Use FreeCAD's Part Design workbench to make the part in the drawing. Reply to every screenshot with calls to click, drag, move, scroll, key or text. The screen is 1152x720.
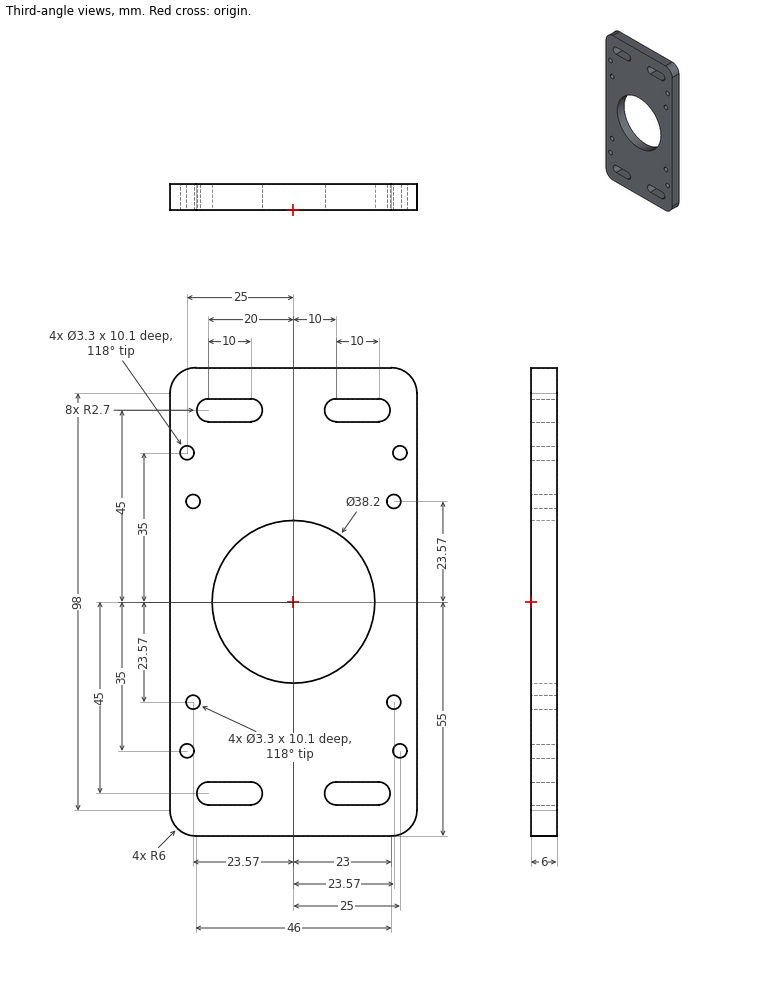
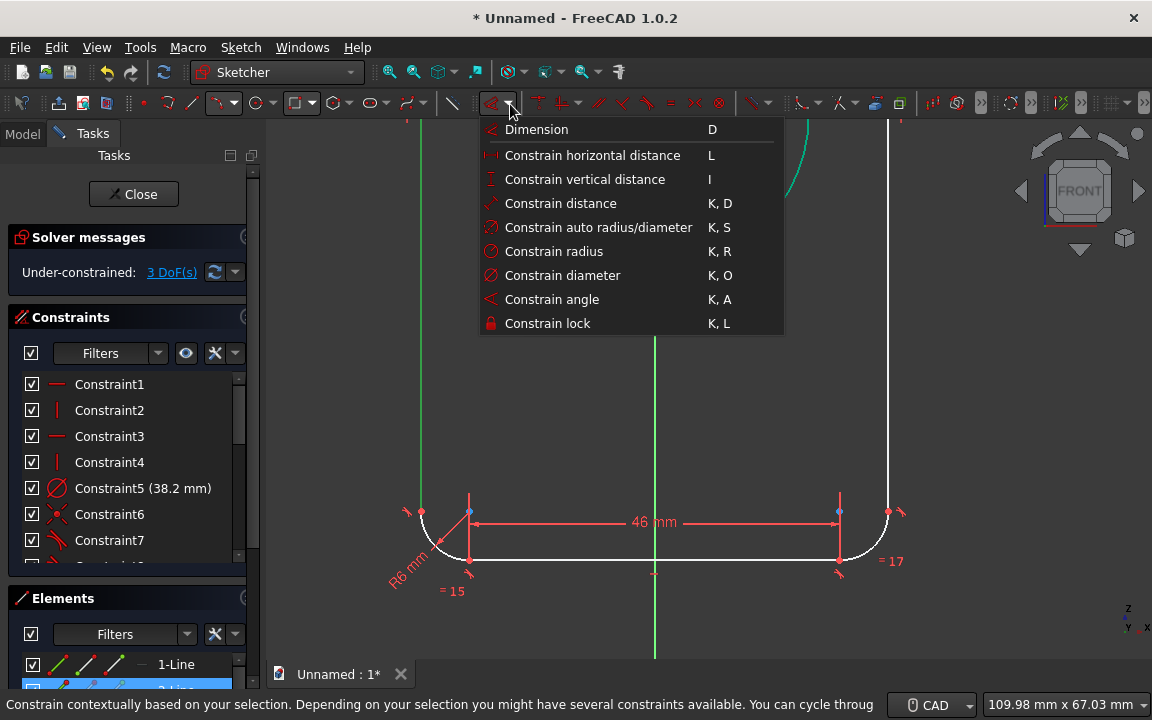
click(632, 179)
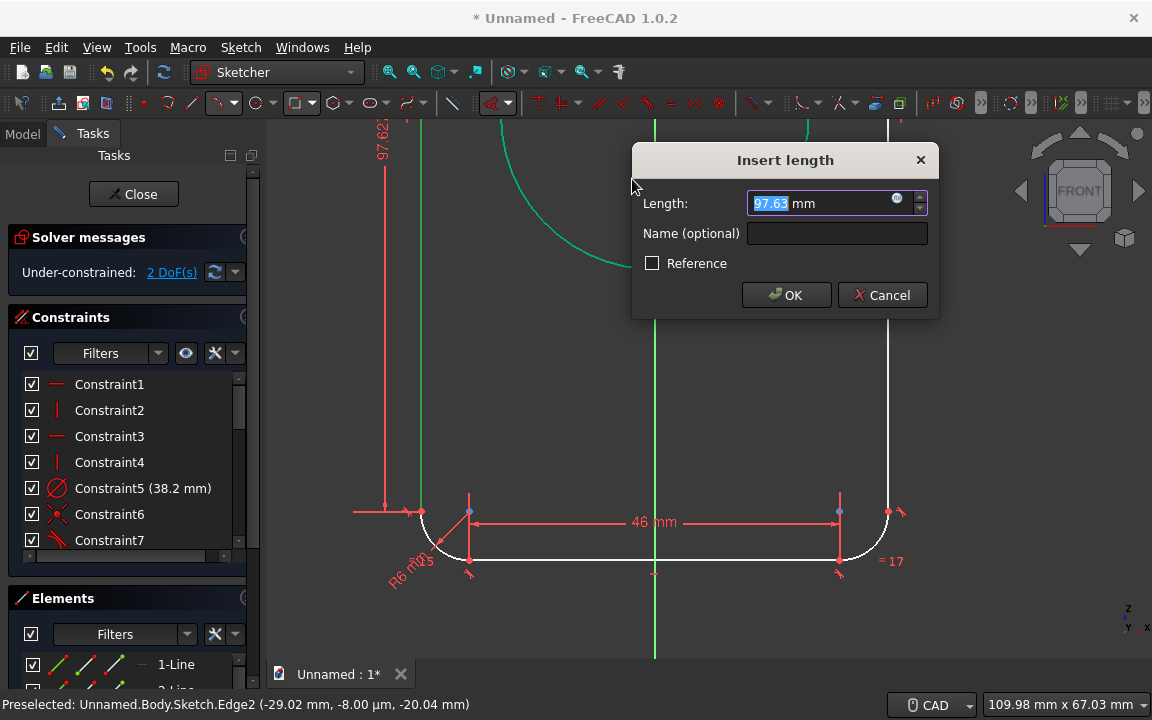
text(98)
key(Return)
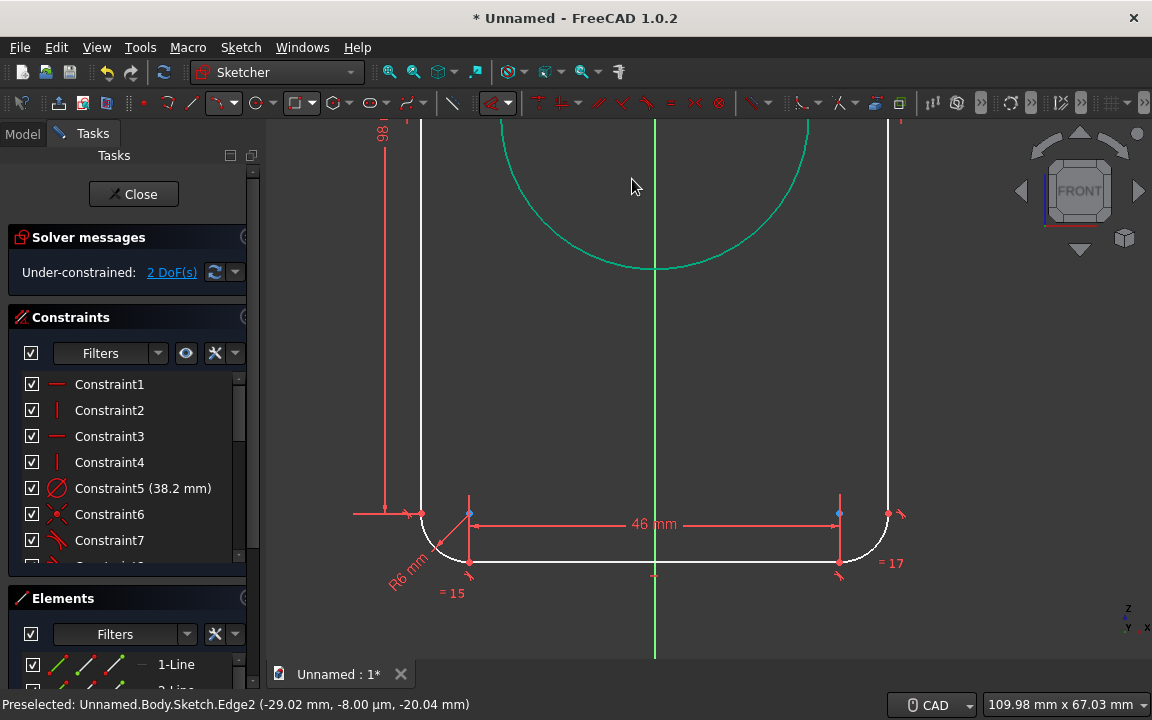
click(840, 562)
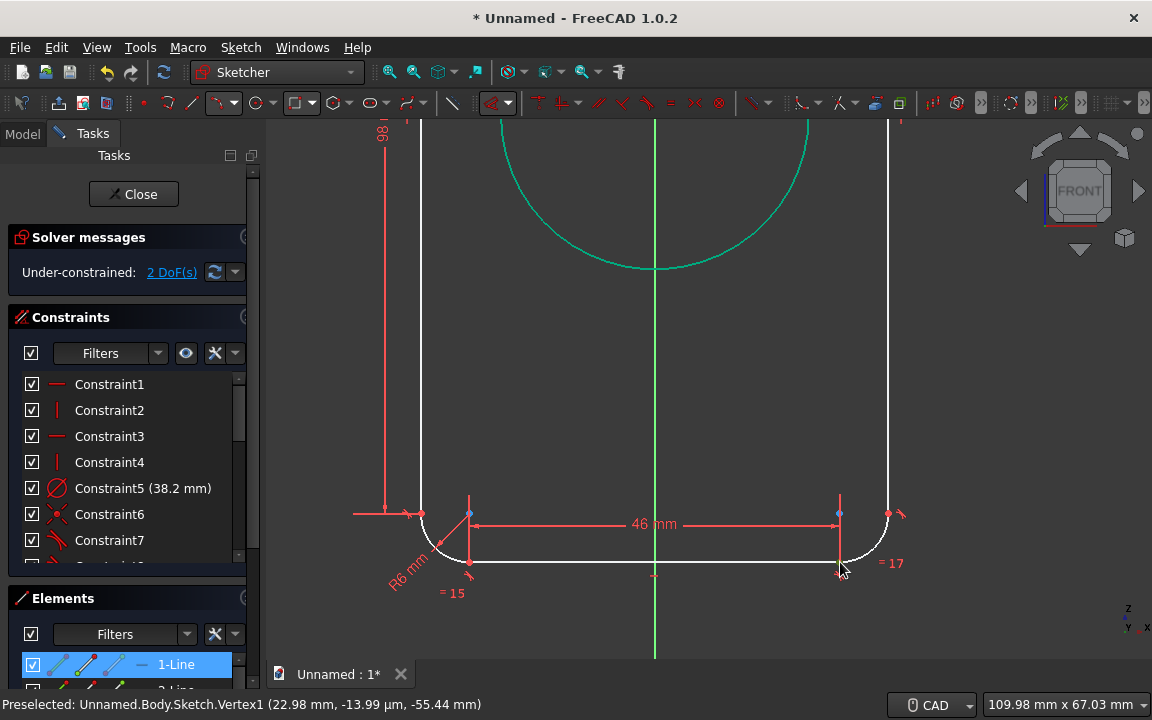
key(l)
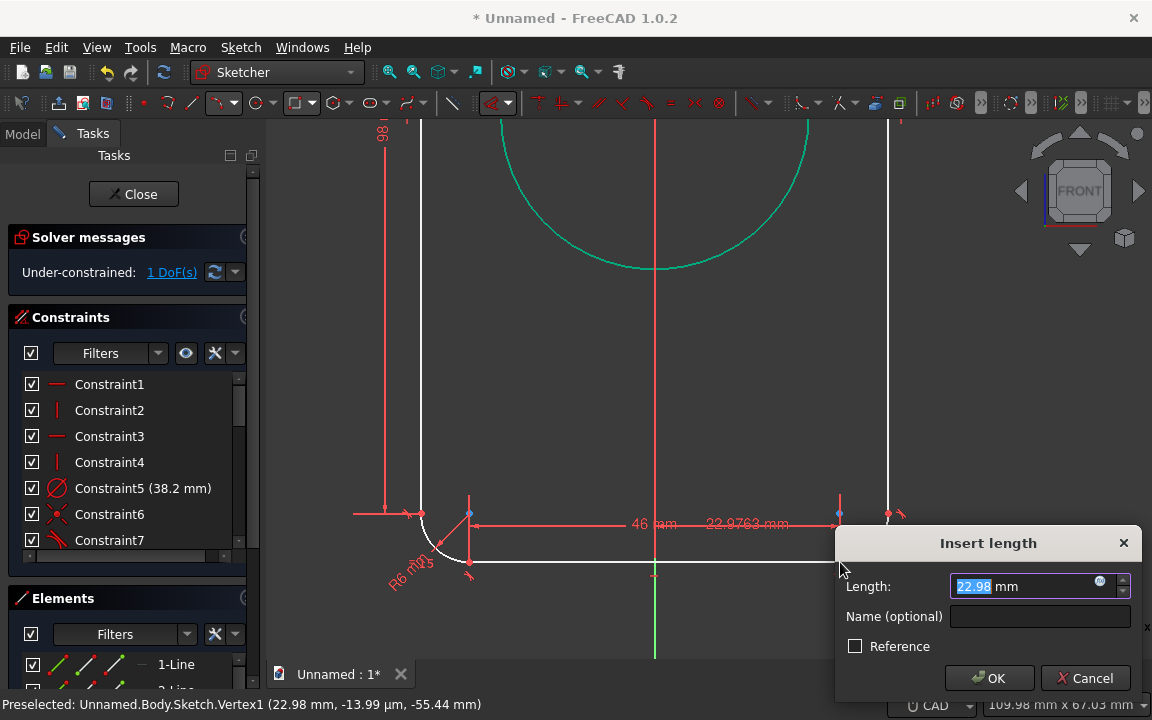
text(23)
key(Return)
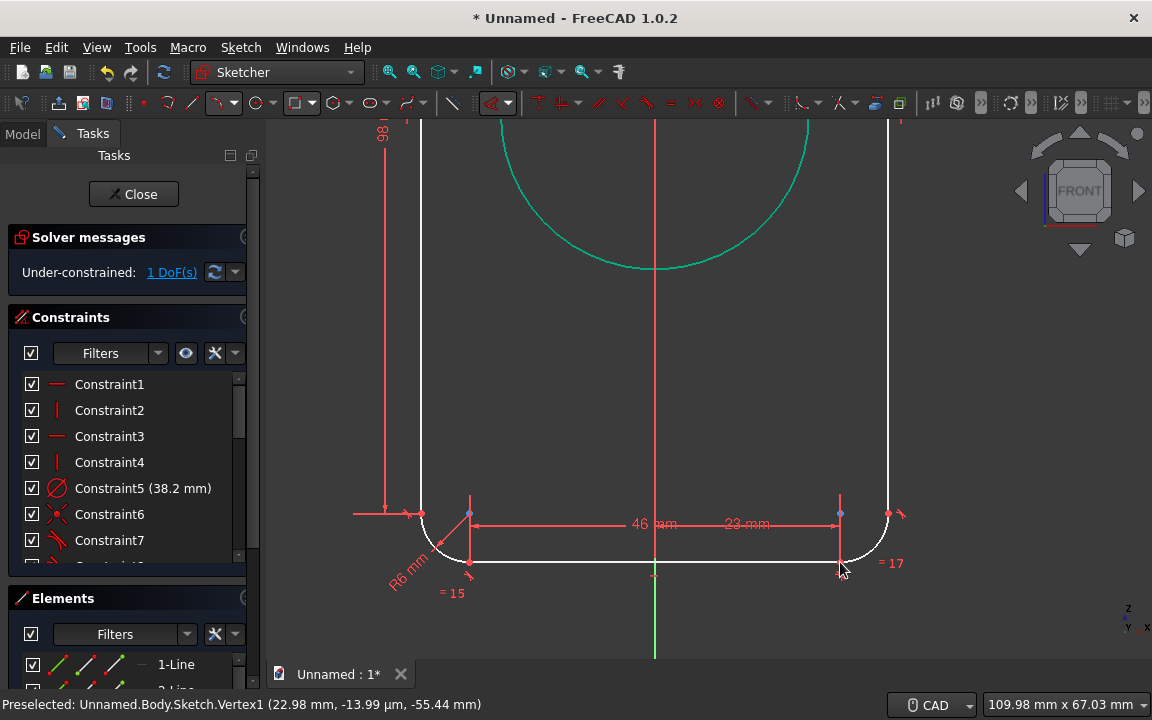
click(840, 562)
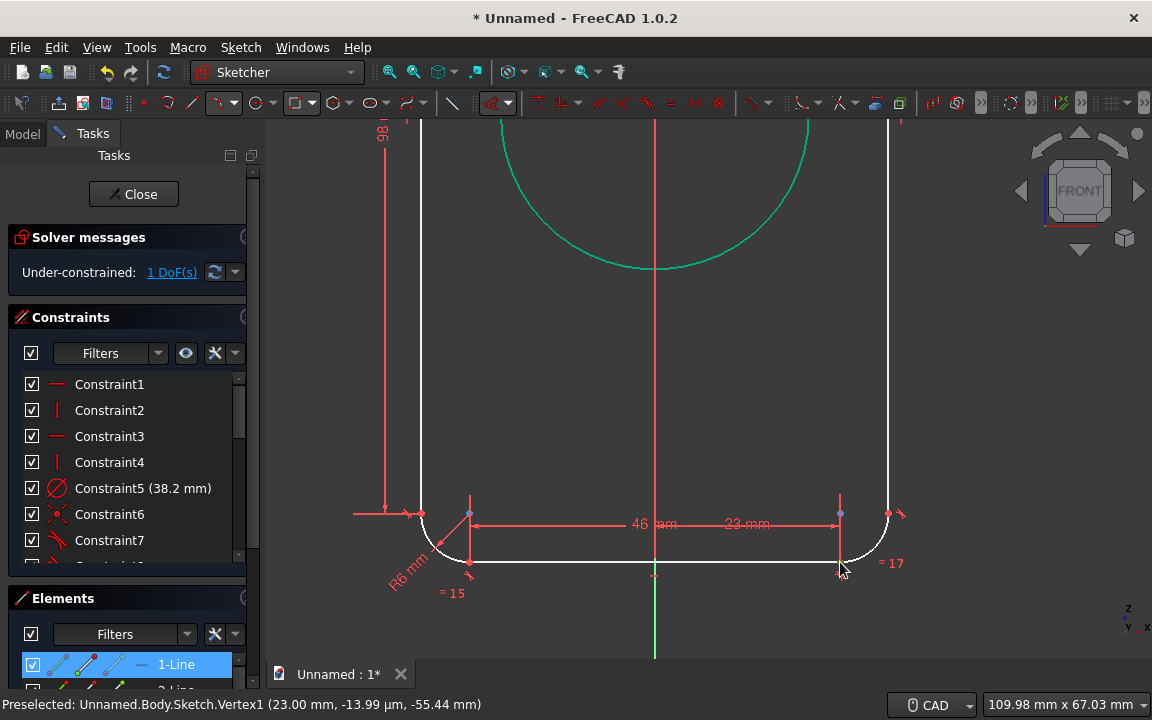
click(510, 104)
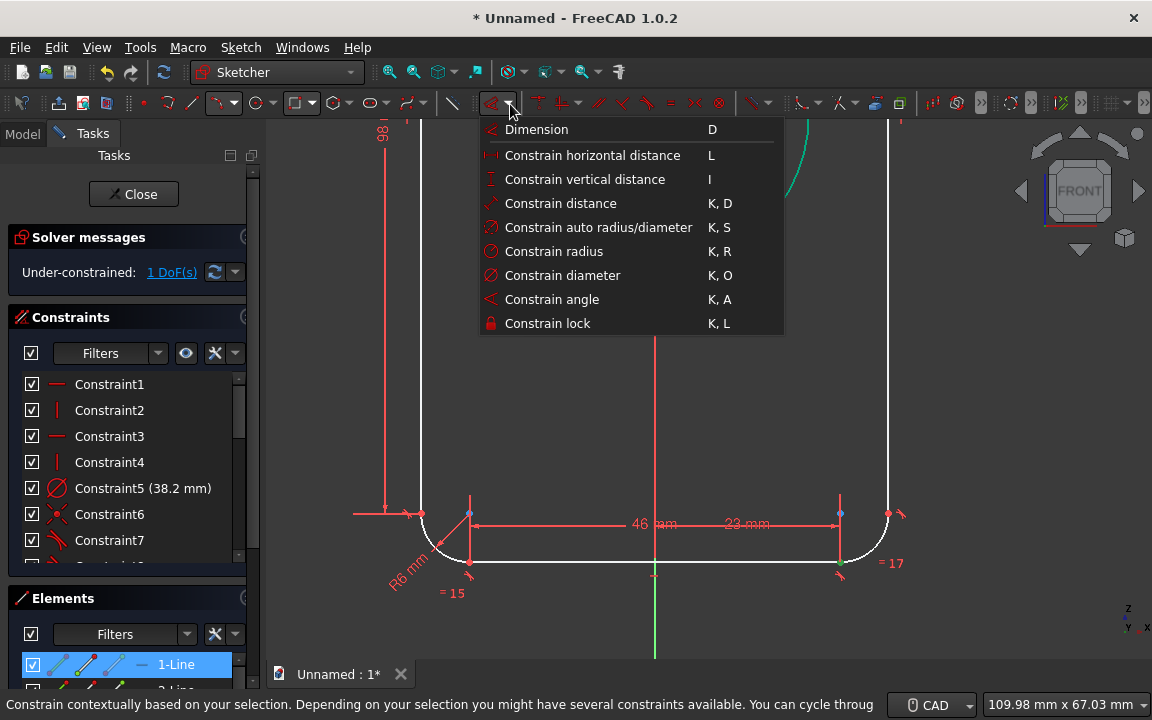
click(632, 179)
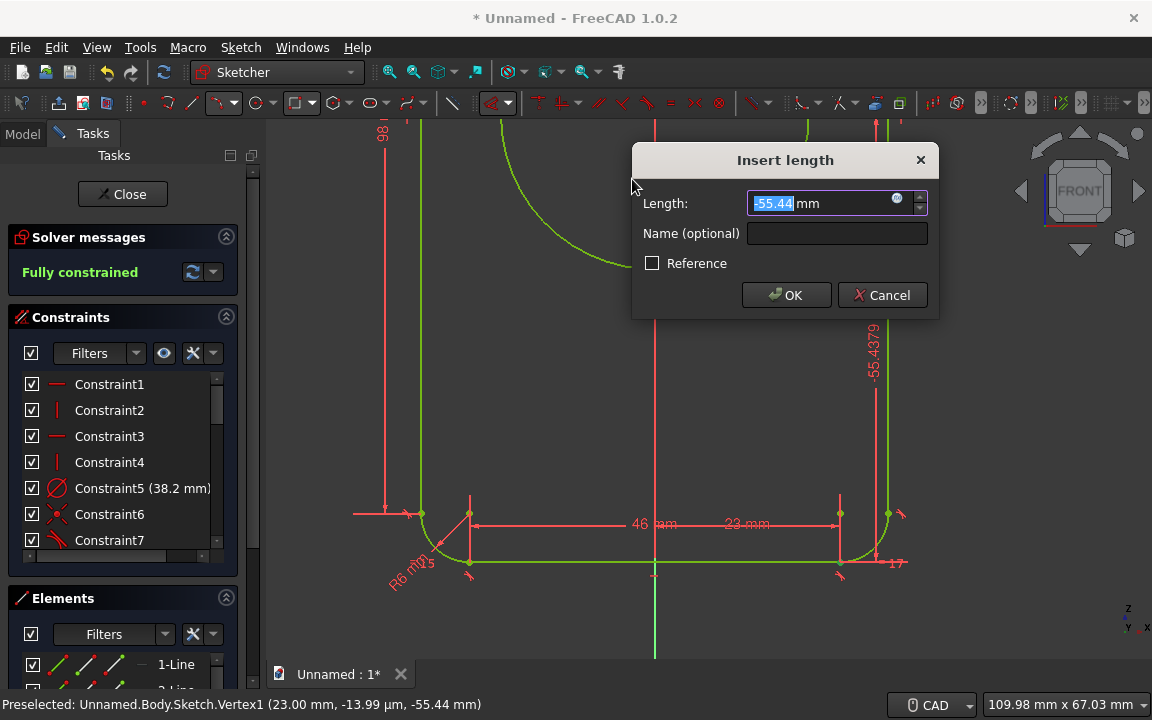
text(-55)
key(Return)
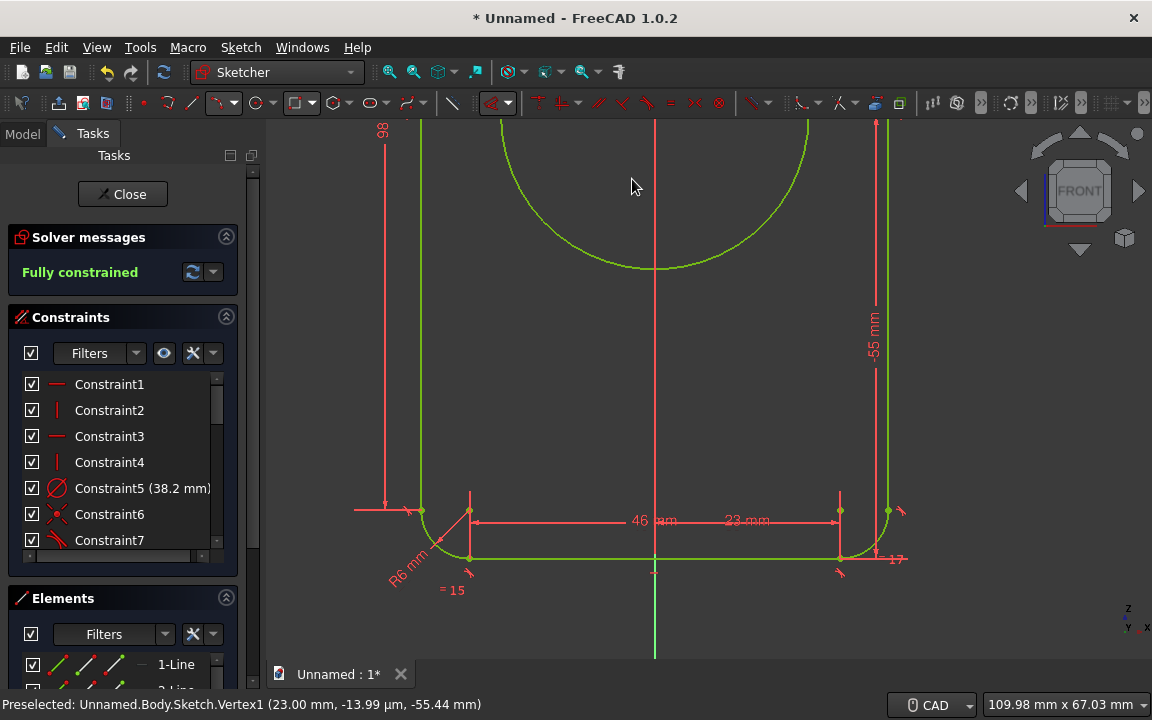
click(123, 194)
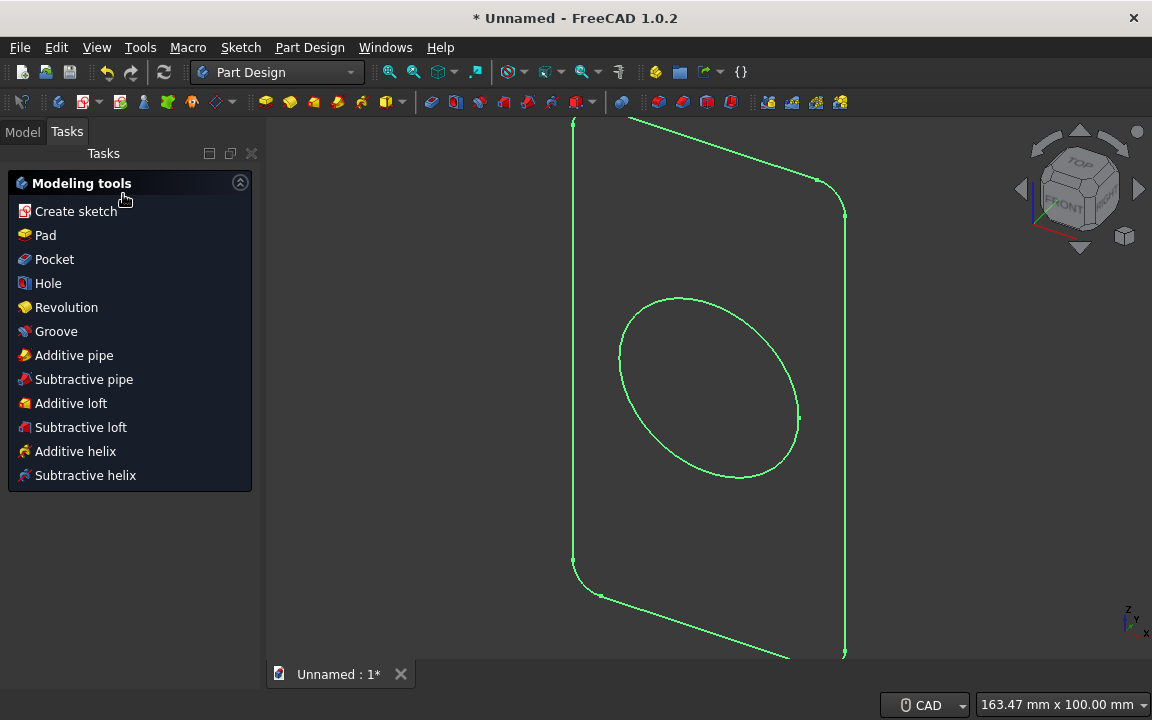
click(266, 102)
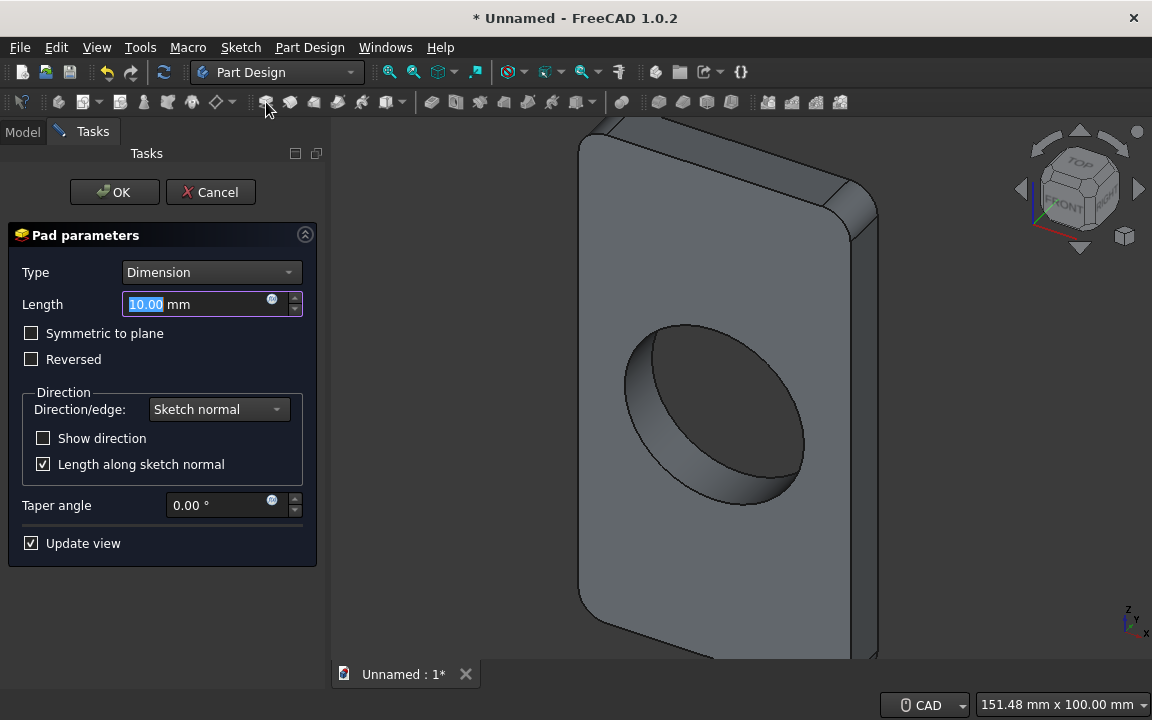
text(6)
key(Tab)